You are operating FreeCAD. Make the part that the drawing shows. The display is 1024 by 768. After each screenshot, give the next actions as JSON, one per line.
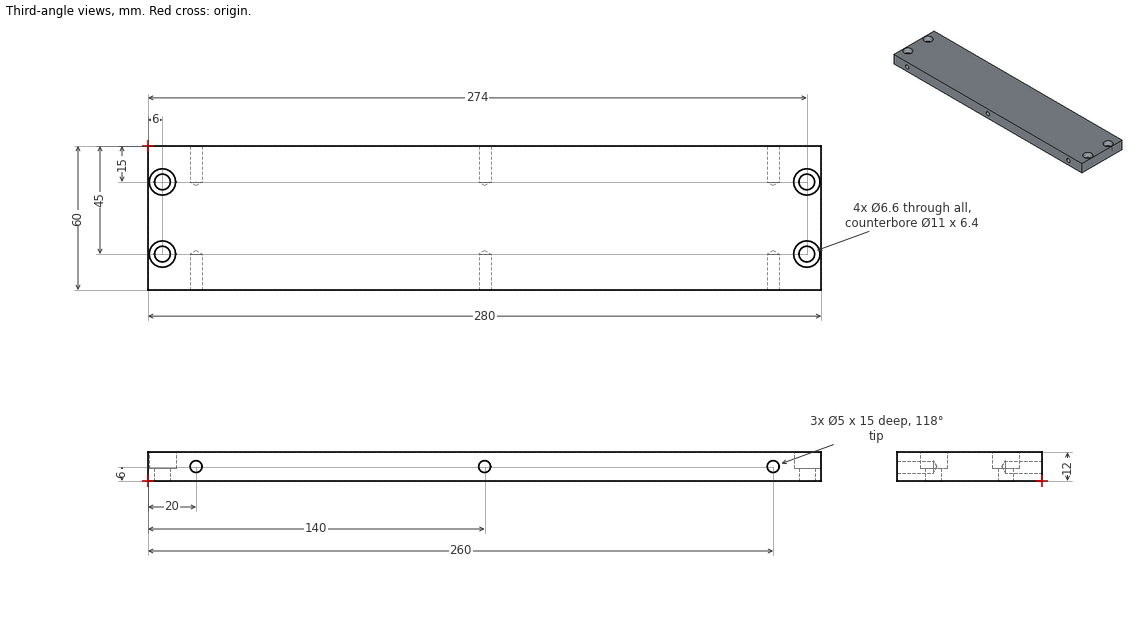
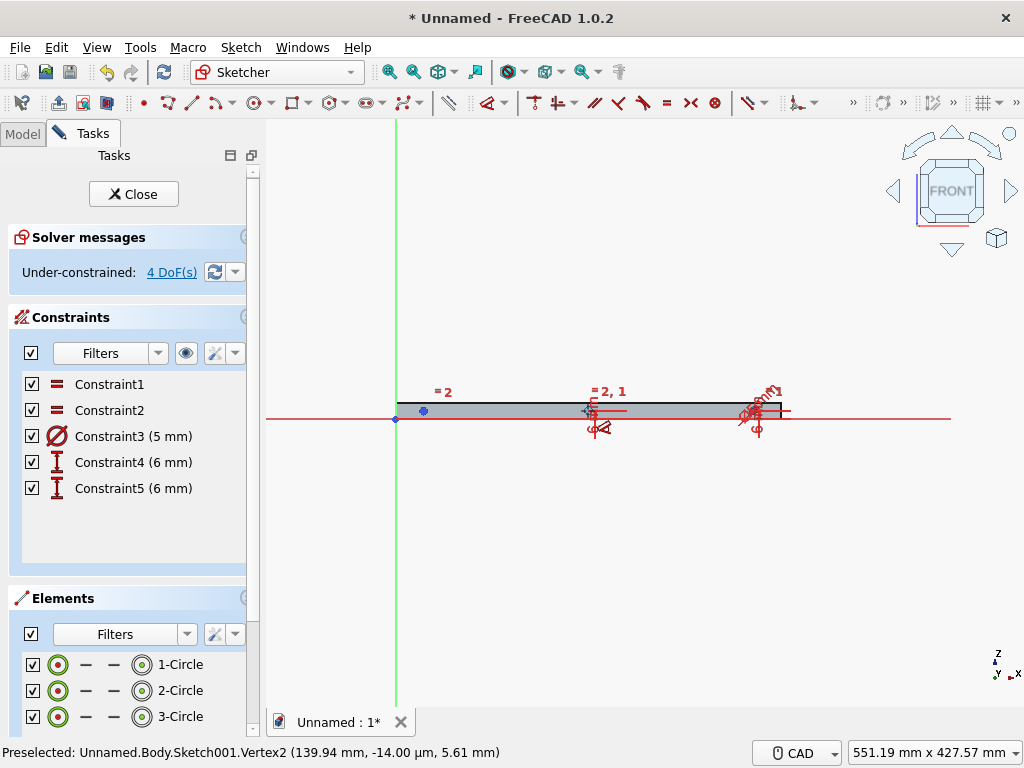
{"action": "scroll", "coordinate": [424, 411], "scroll_direction": "up", "scroll_amount": 8}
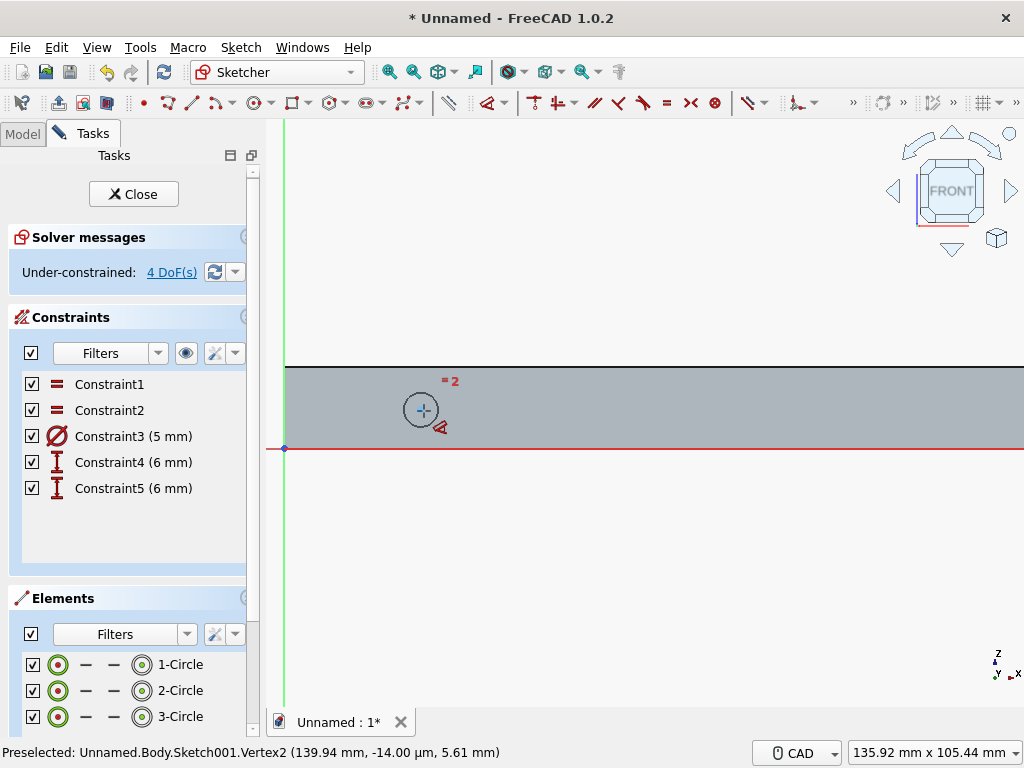
{"action": "left_click", "coordinate": [421, 410]}
{"action": "left_click", "coordinate": [455, 429]}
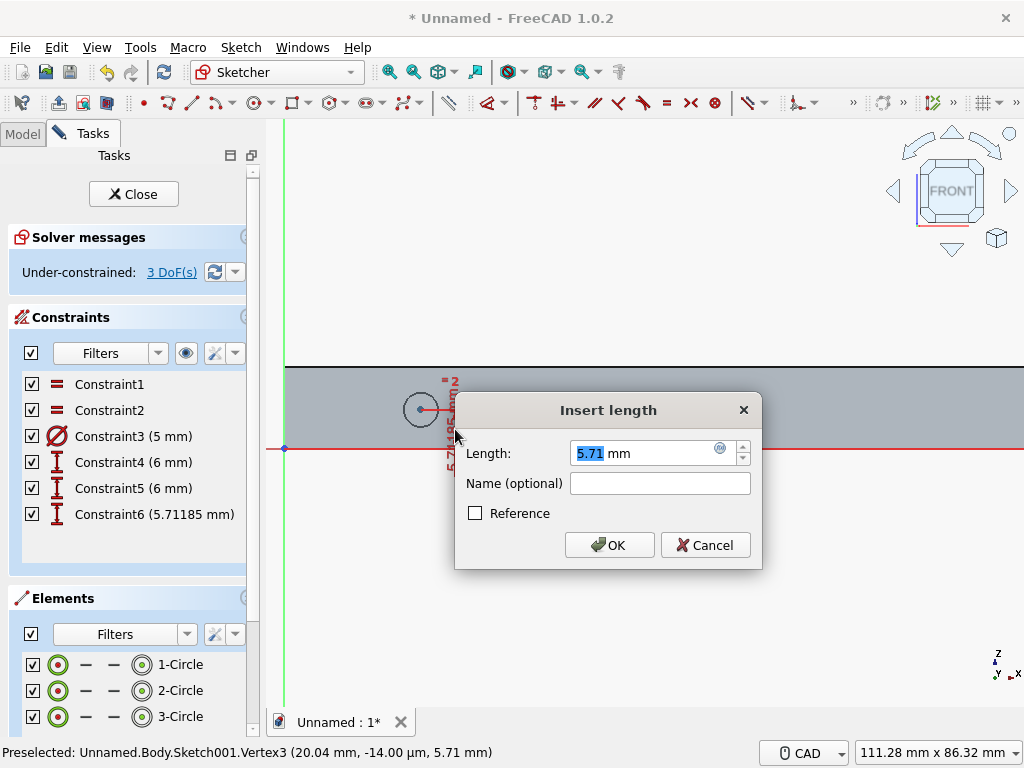
{"action": "type", "text": "6"}
{"action": "key", "text": "Return"}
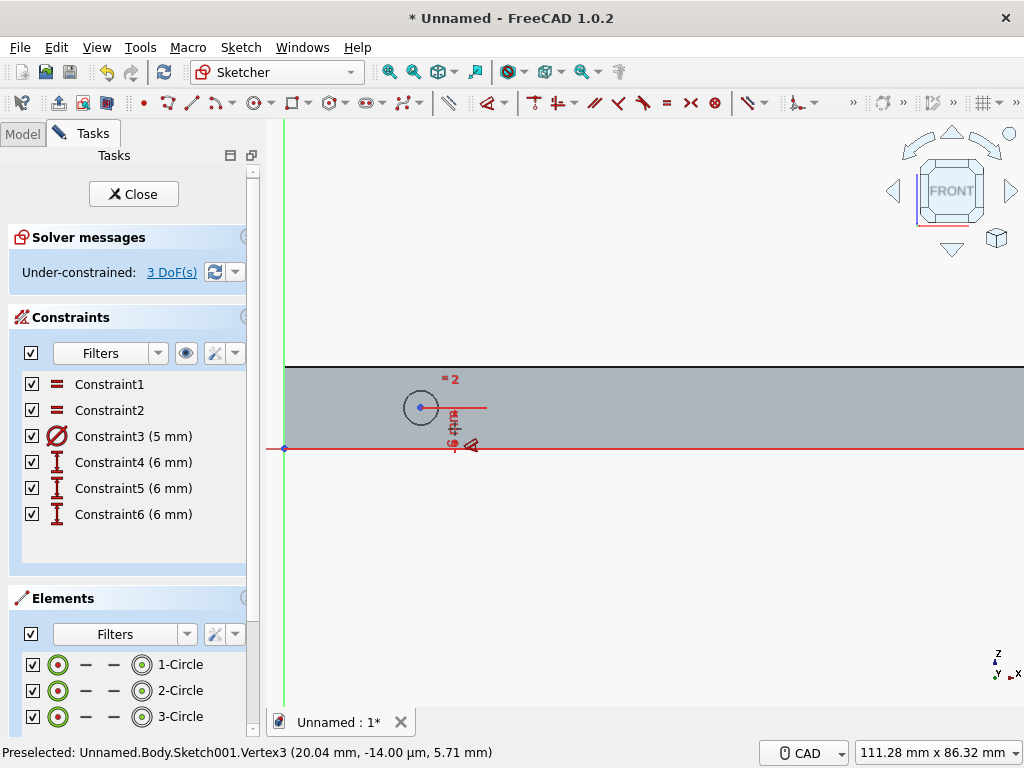
{"action": "scroll", "coordinate": [424, 411], "scroll_direction": "down", "scroll_amount": 8}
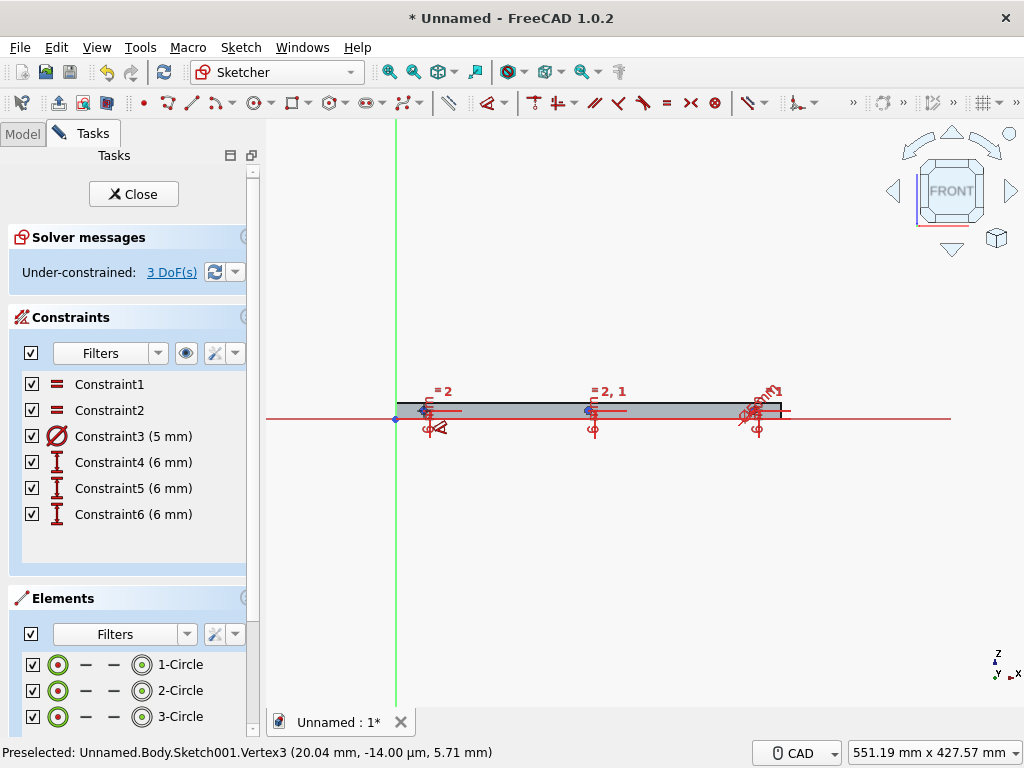
{"action": "scroll", "coordinate": [424, 411], "scroll_direction": "up", "scroll_amount": 2}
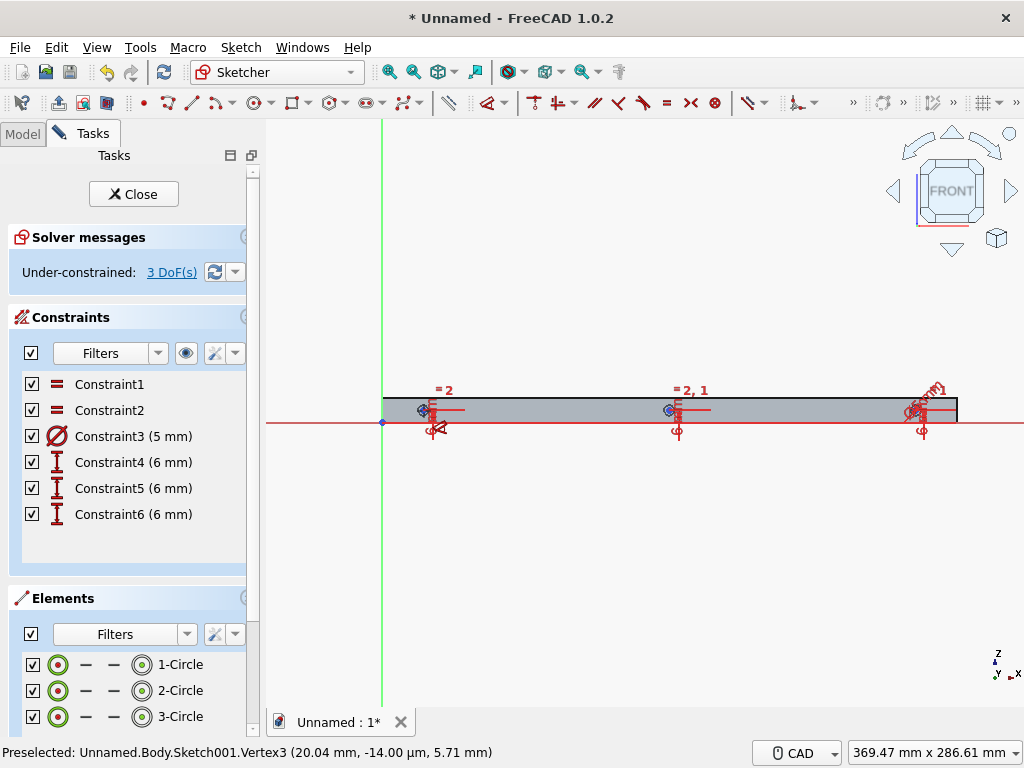
{"action": "left_click", "coordinate": [423, 410]}
{"action": "left_click", "coordinate": [403, 457]}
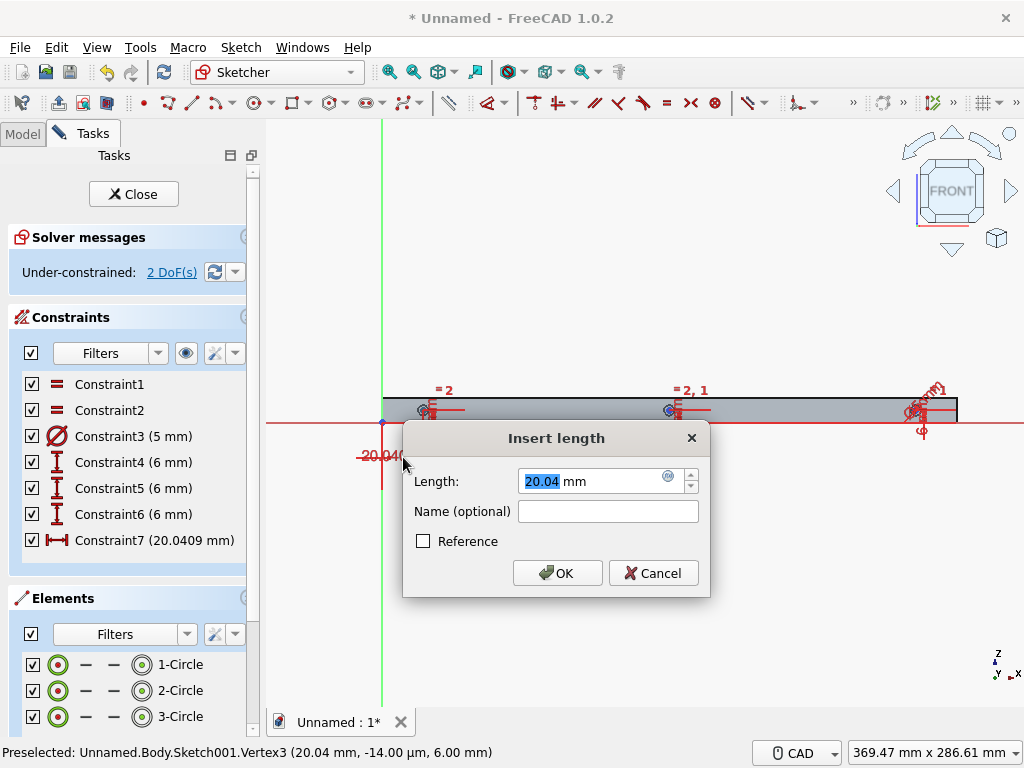
{"action": "type", "text": "20"}
{"action": "key", "text": "Return"}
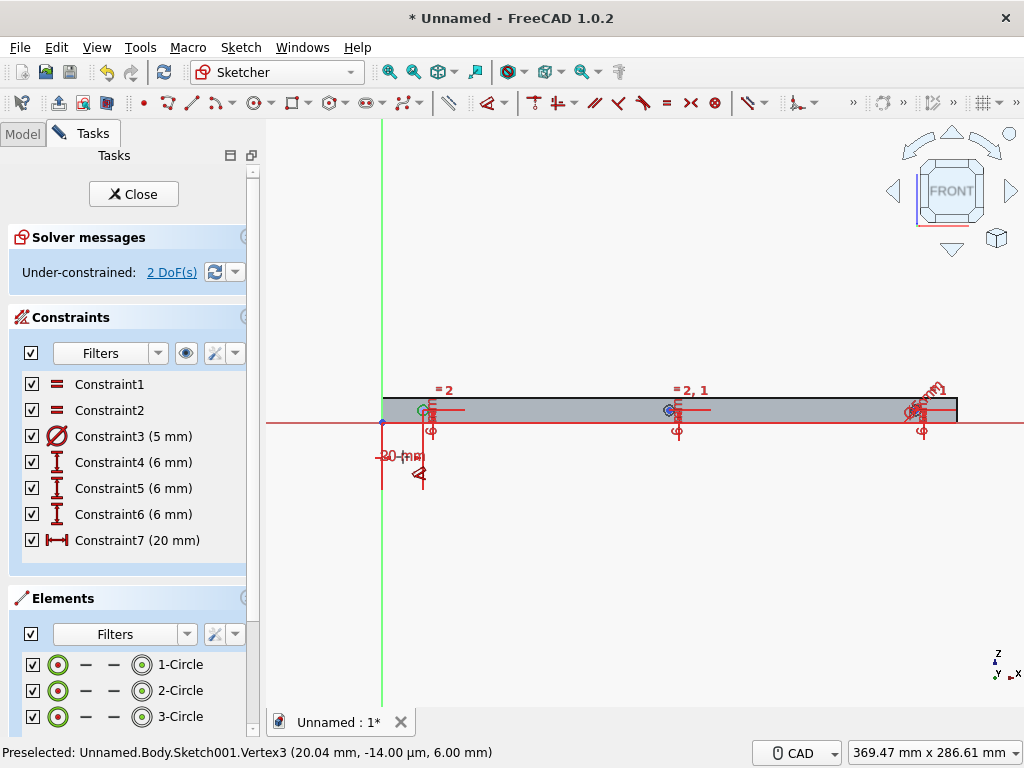
{"action": "scroll", "coordinate": [424, 411], "scroll_direction": "down", "scroll_amount": 2}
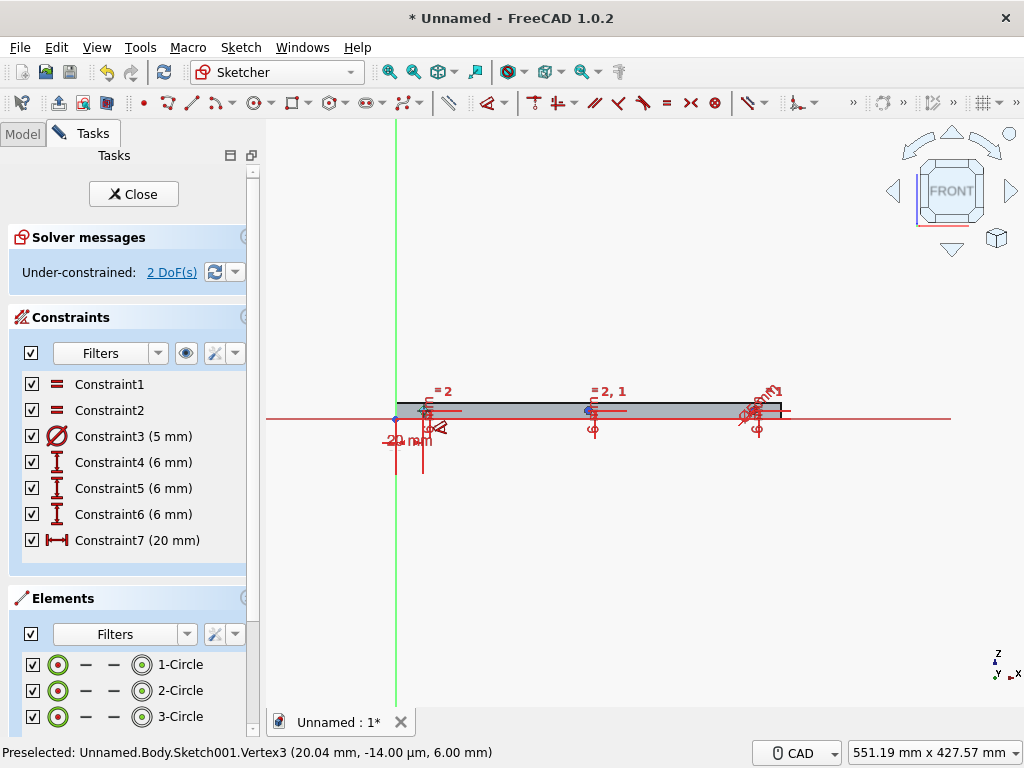
{"action": "left_click", "coordinate": [754, 411]}
{"action": "left_click", "coordinate": [575, 453]}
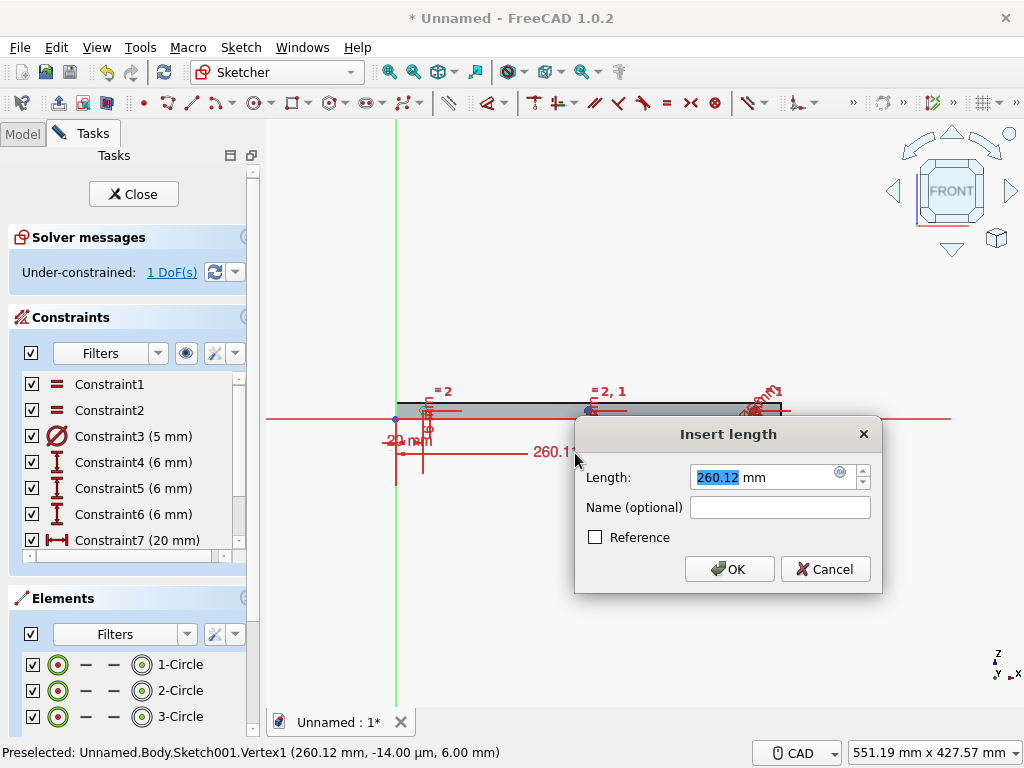
{"action": "type", "text": "260"}
{"action": "key", "text": "Return"}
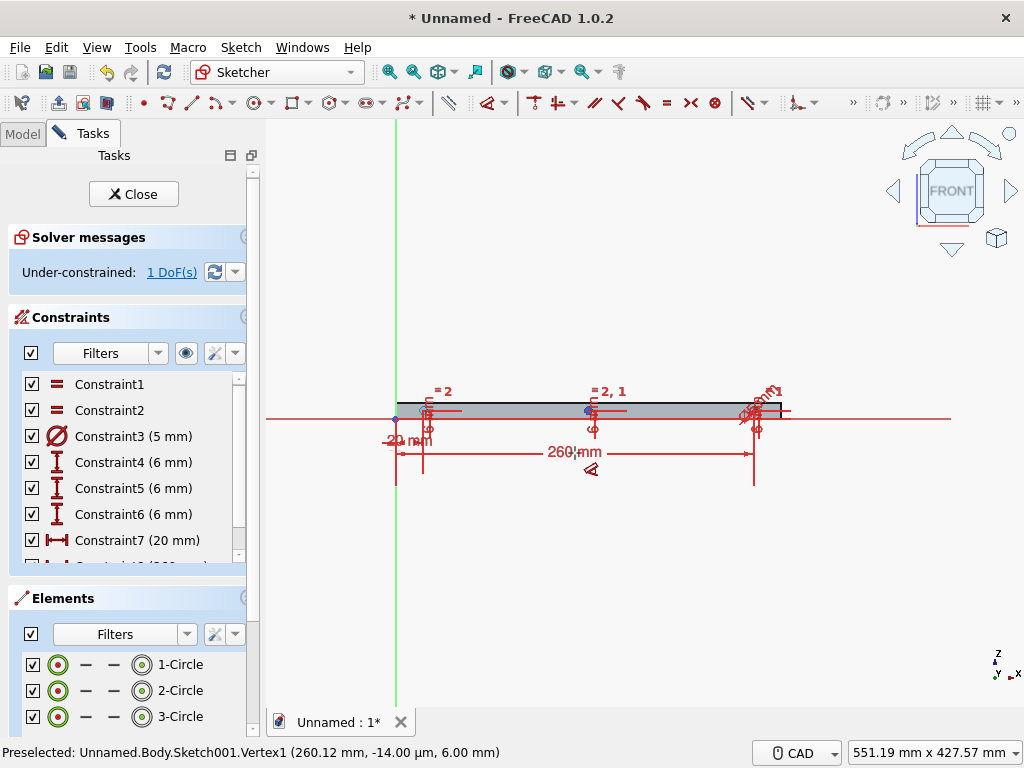
{"action": "left_click", "coordinate": [588, 411]}
{"action": "left_click", "coordinate": [492, 453]}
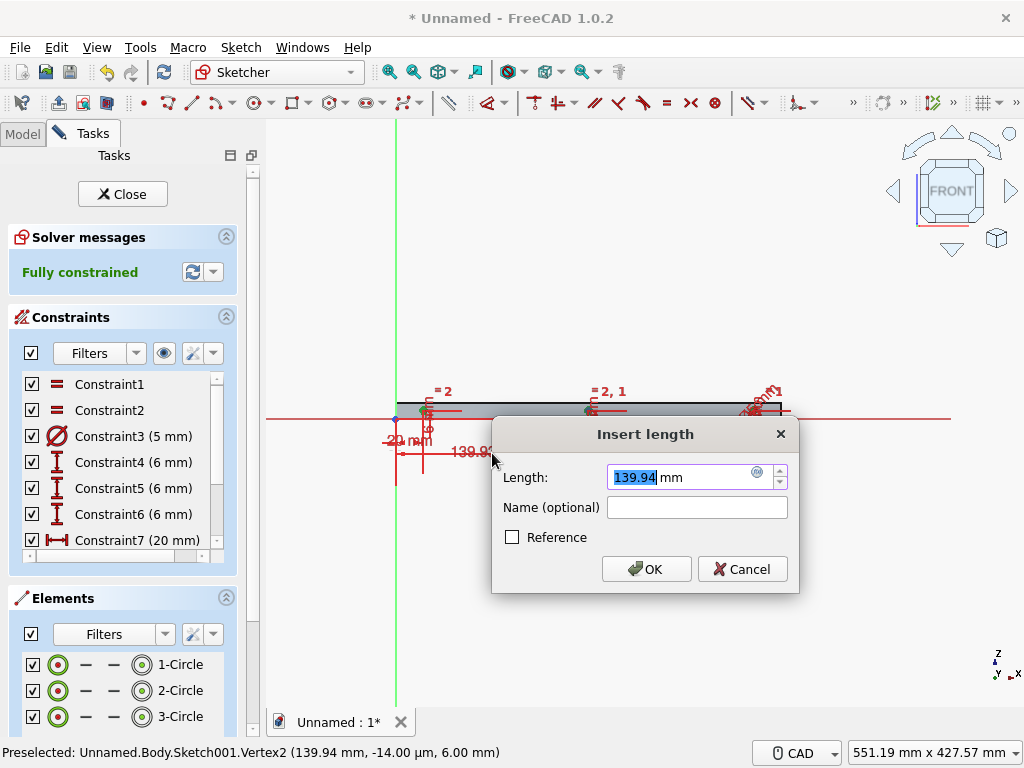
{"action": "type", "text": "140"}
{"action": "key", "text": "Return"}
{"action": "key", "text": "Escape"}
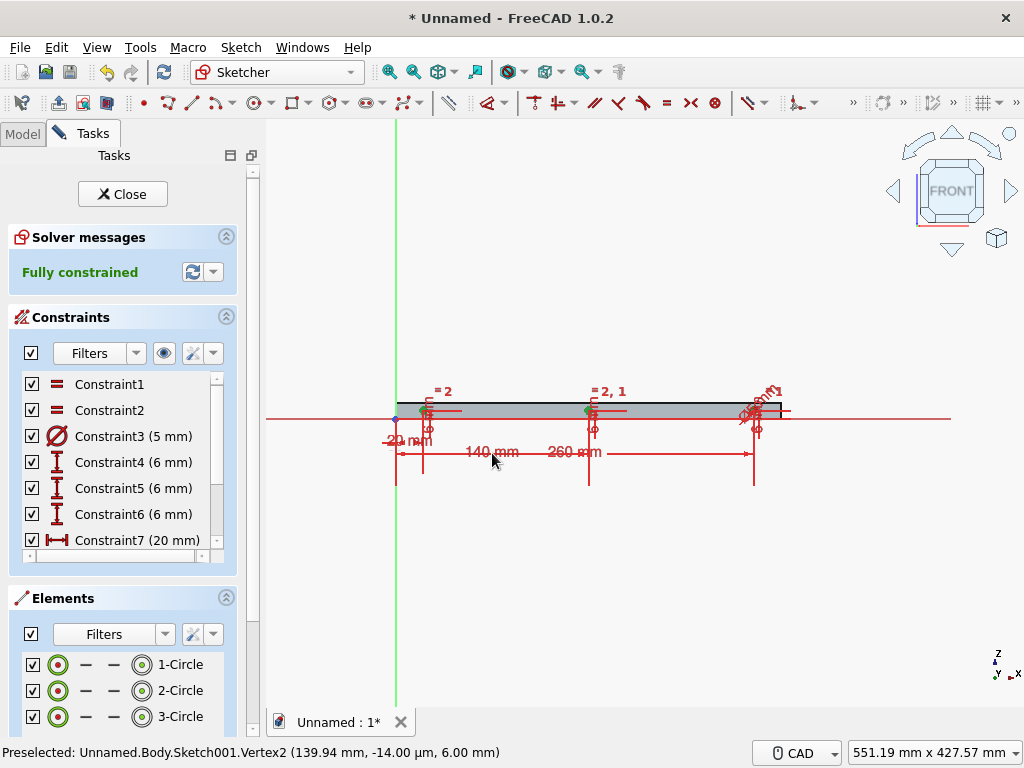
{"action": "left_click", "coordinate": [123, 194]}